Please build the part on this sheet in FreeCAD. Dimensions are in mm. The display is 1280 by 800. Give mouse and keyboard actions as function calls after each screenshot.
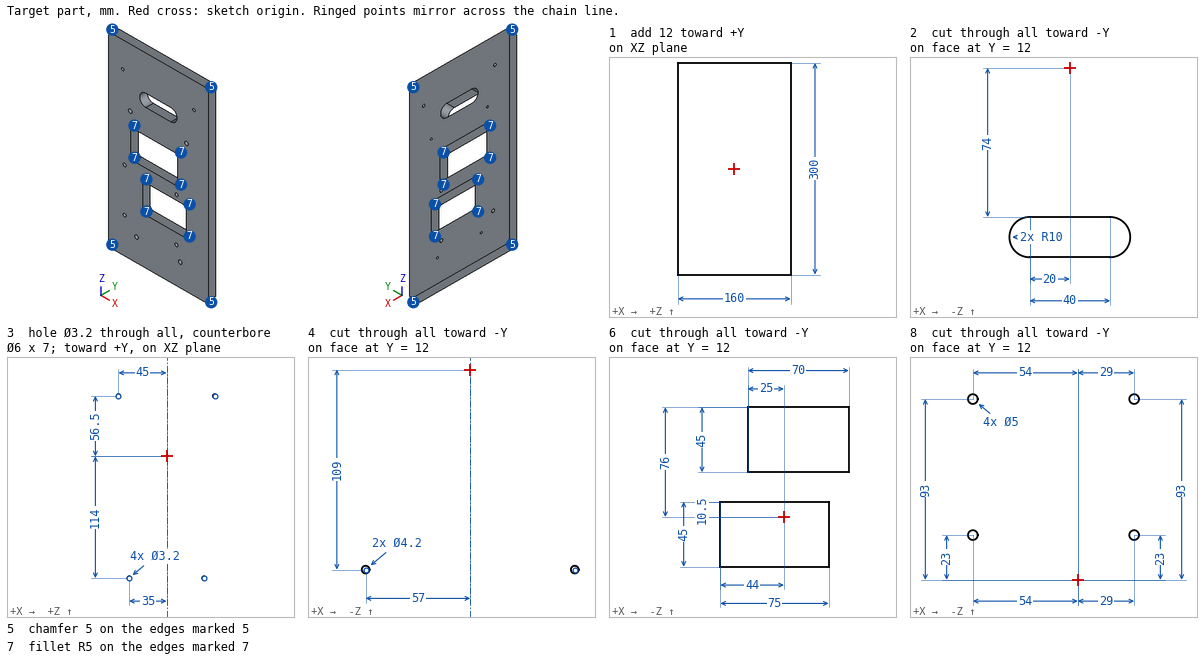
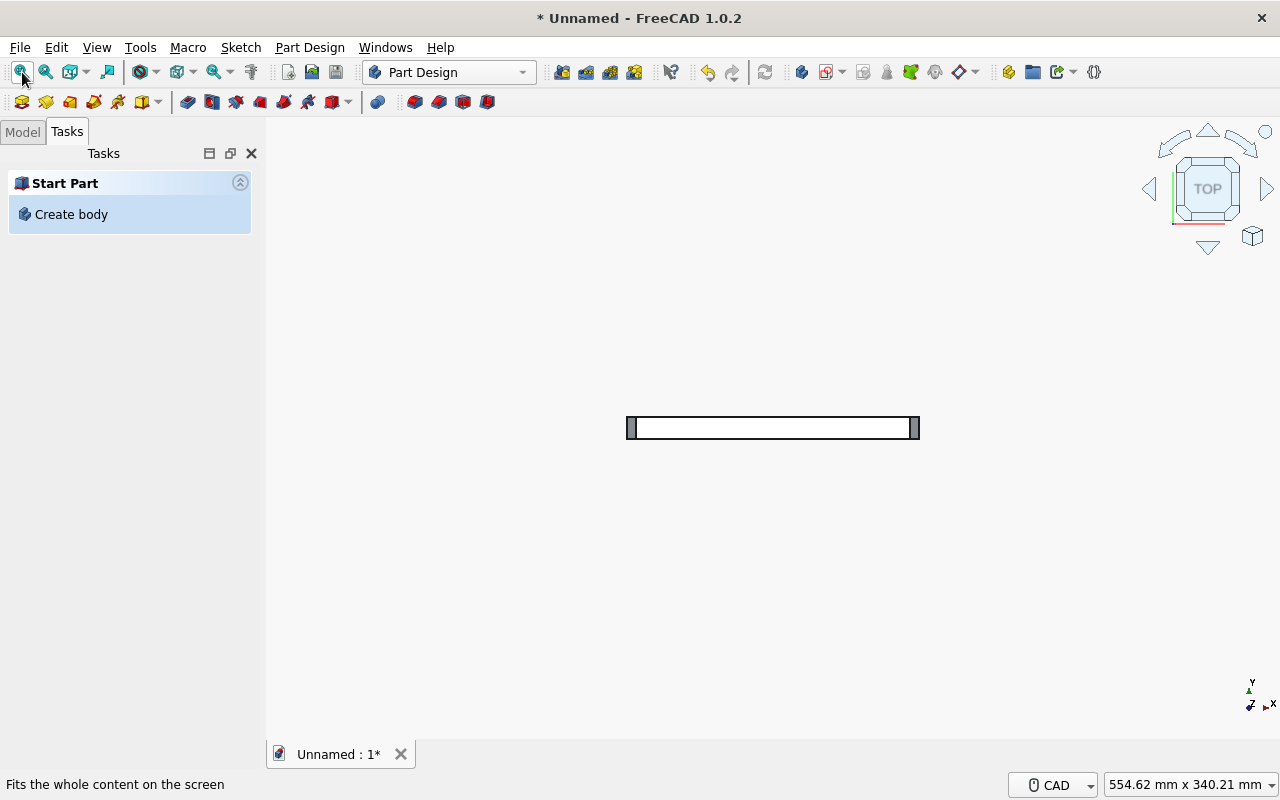
click(22, 72)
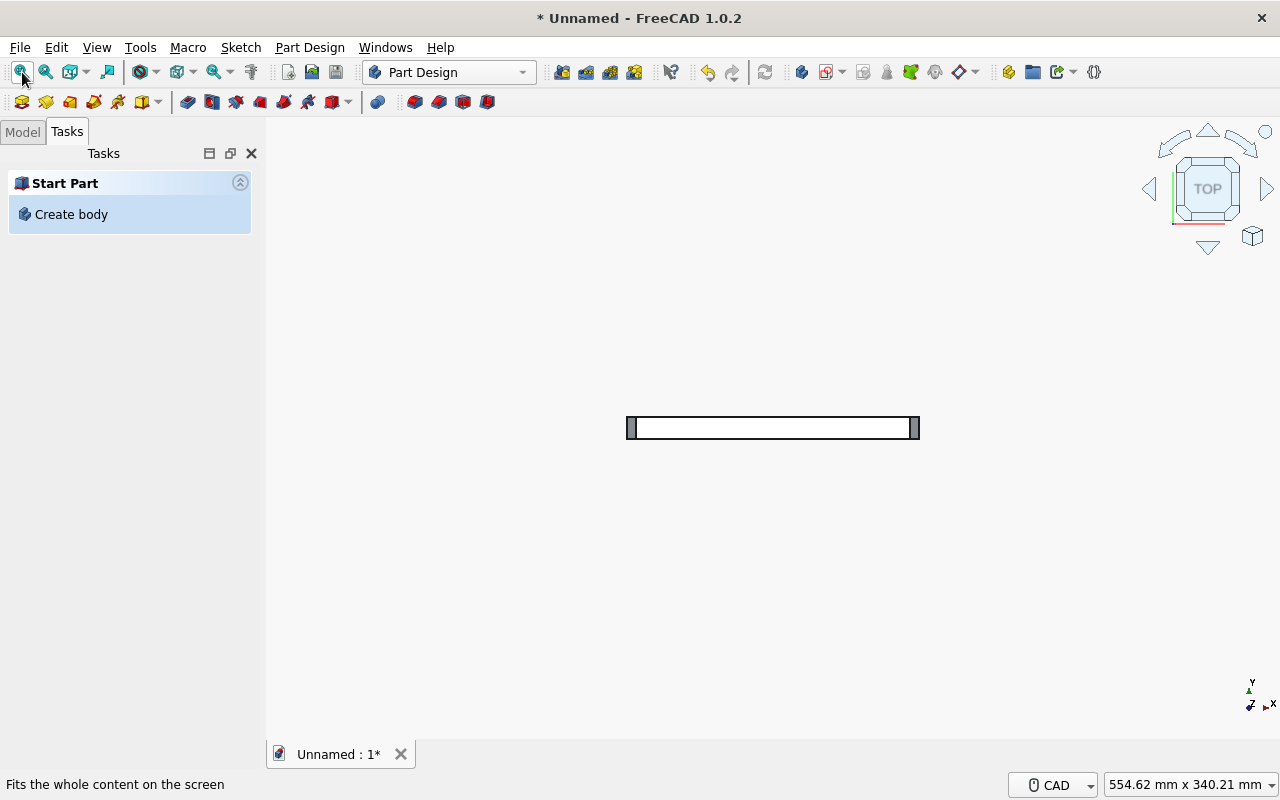
scroll(830, 427, up, 4)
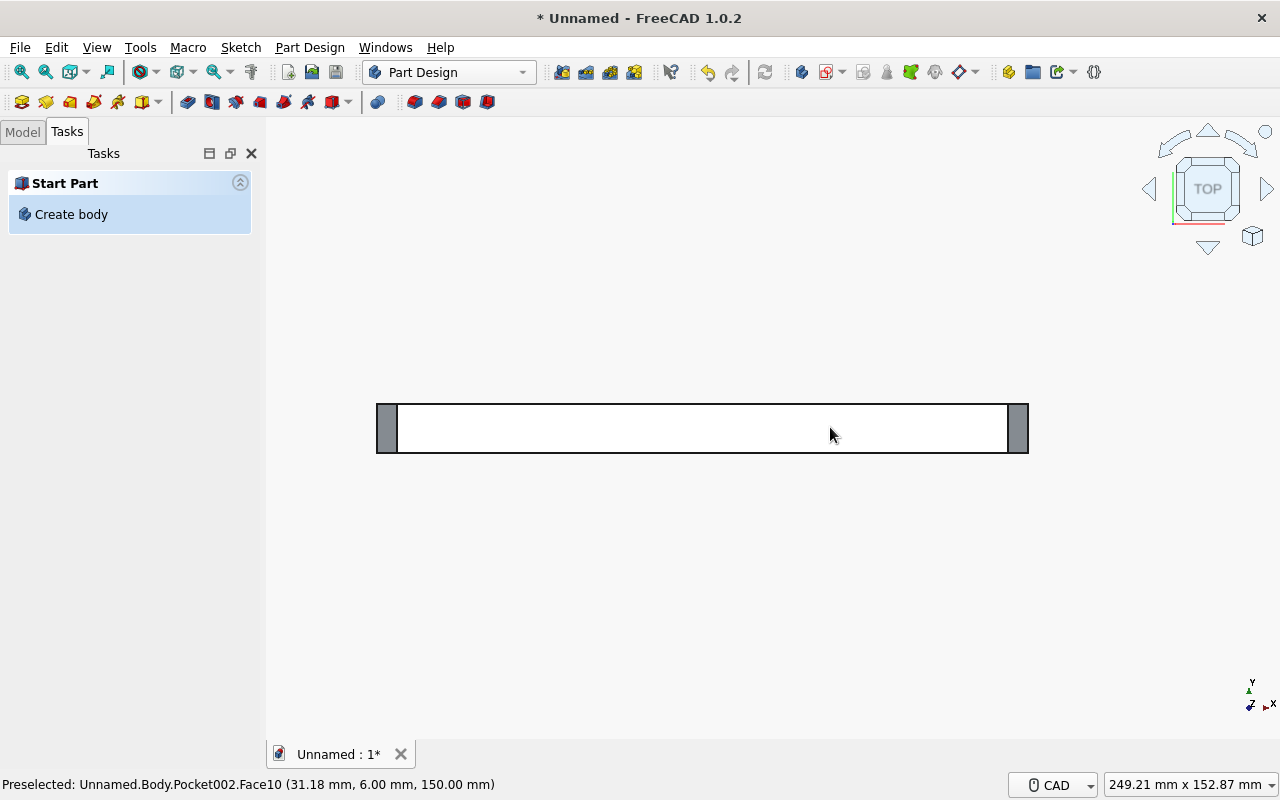
click(22, 72)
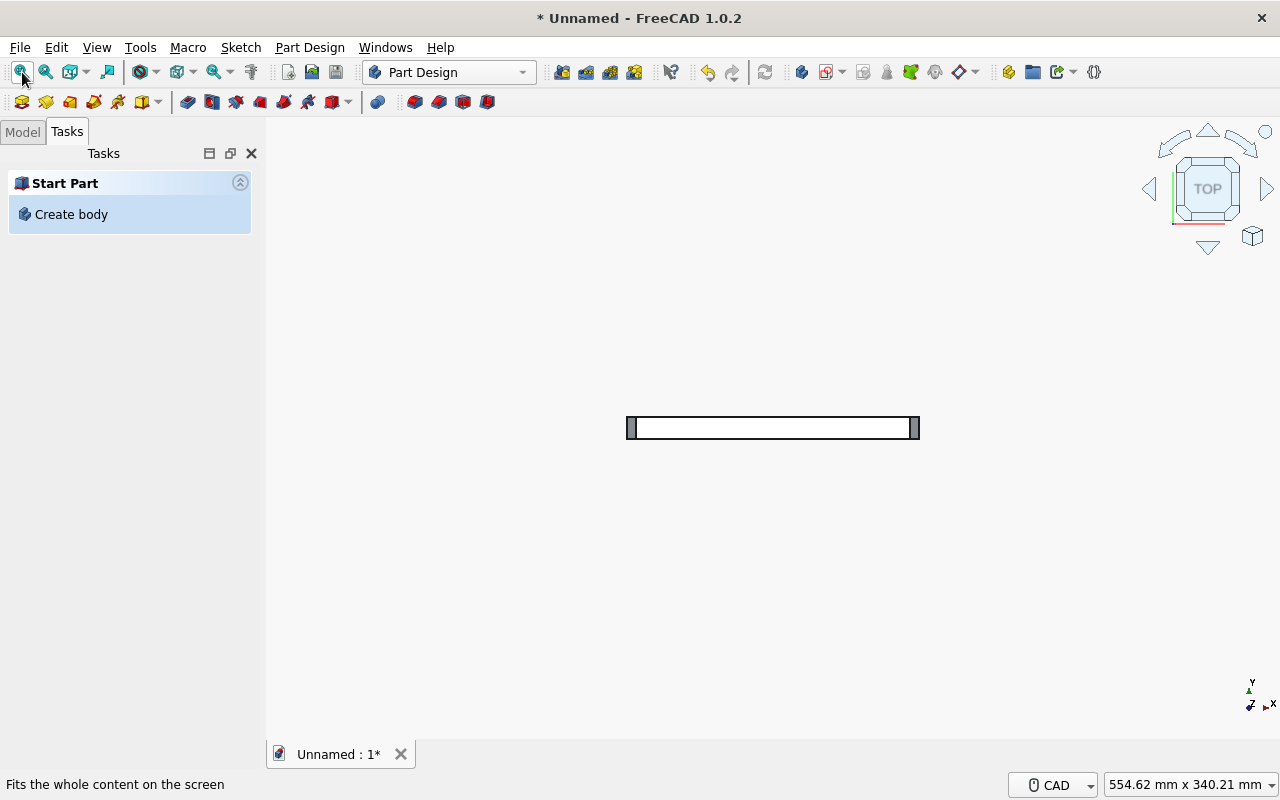
key(1)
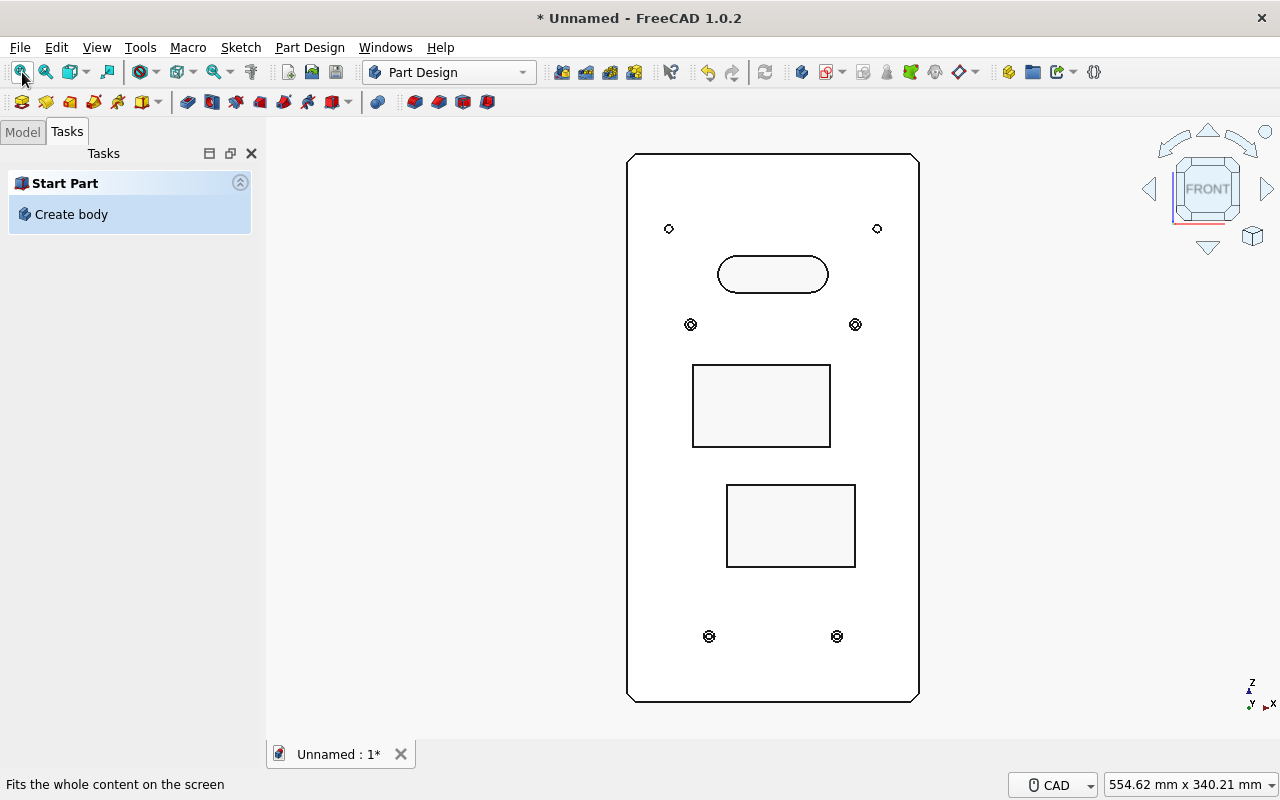
scroll(830, 446, up, 4)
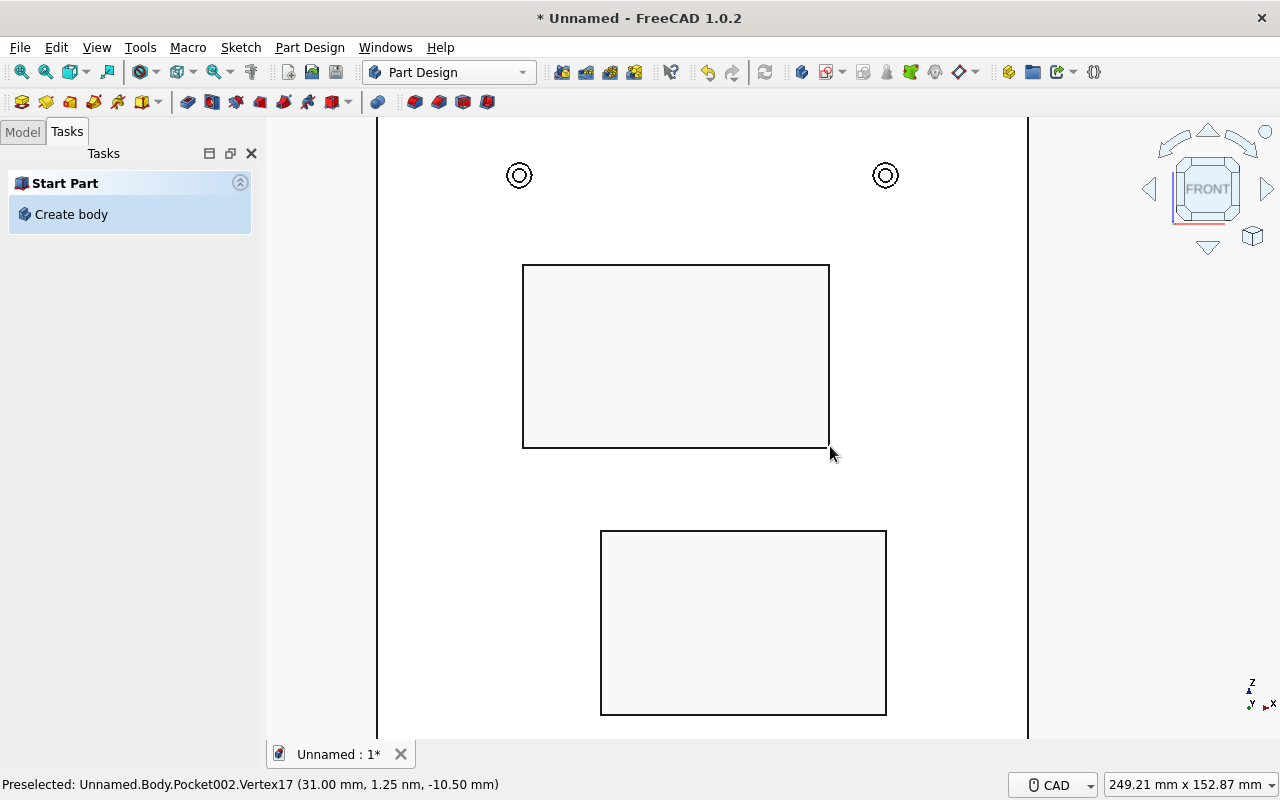
click(22, 72)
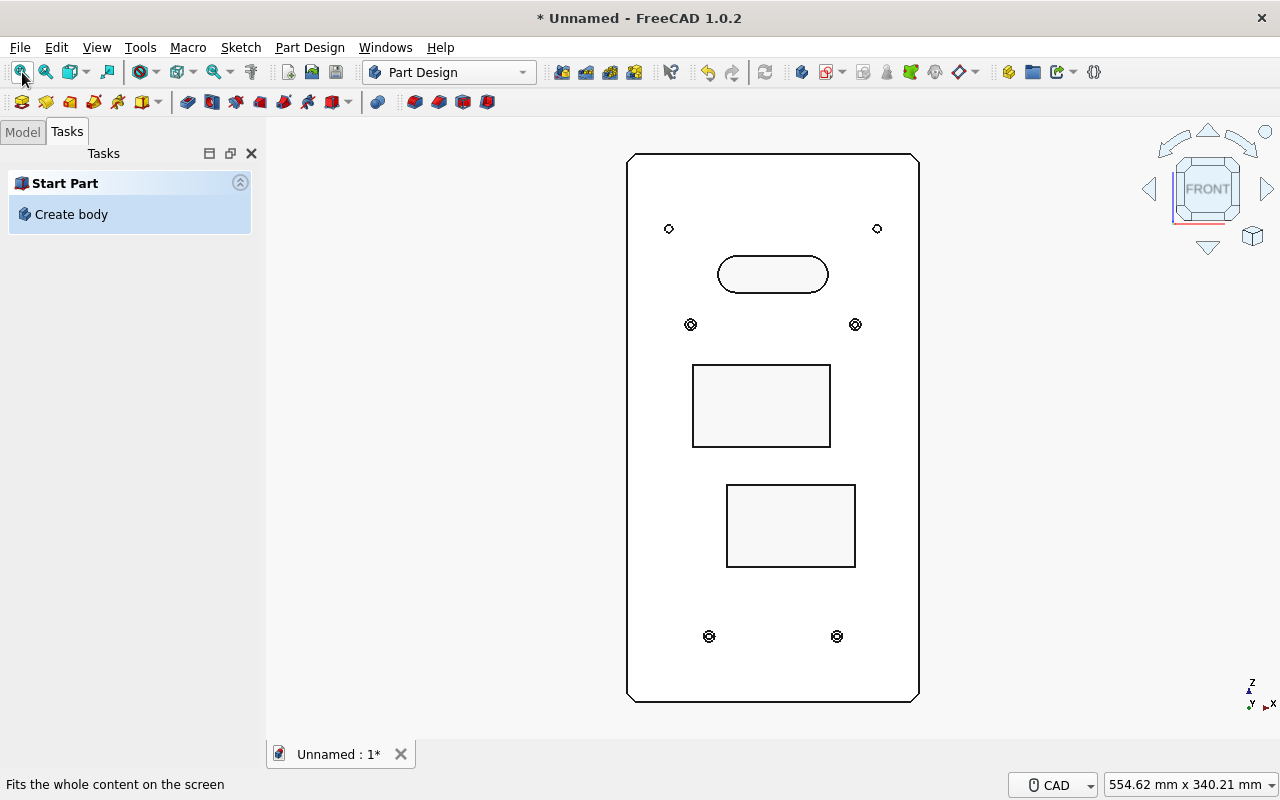
key(3)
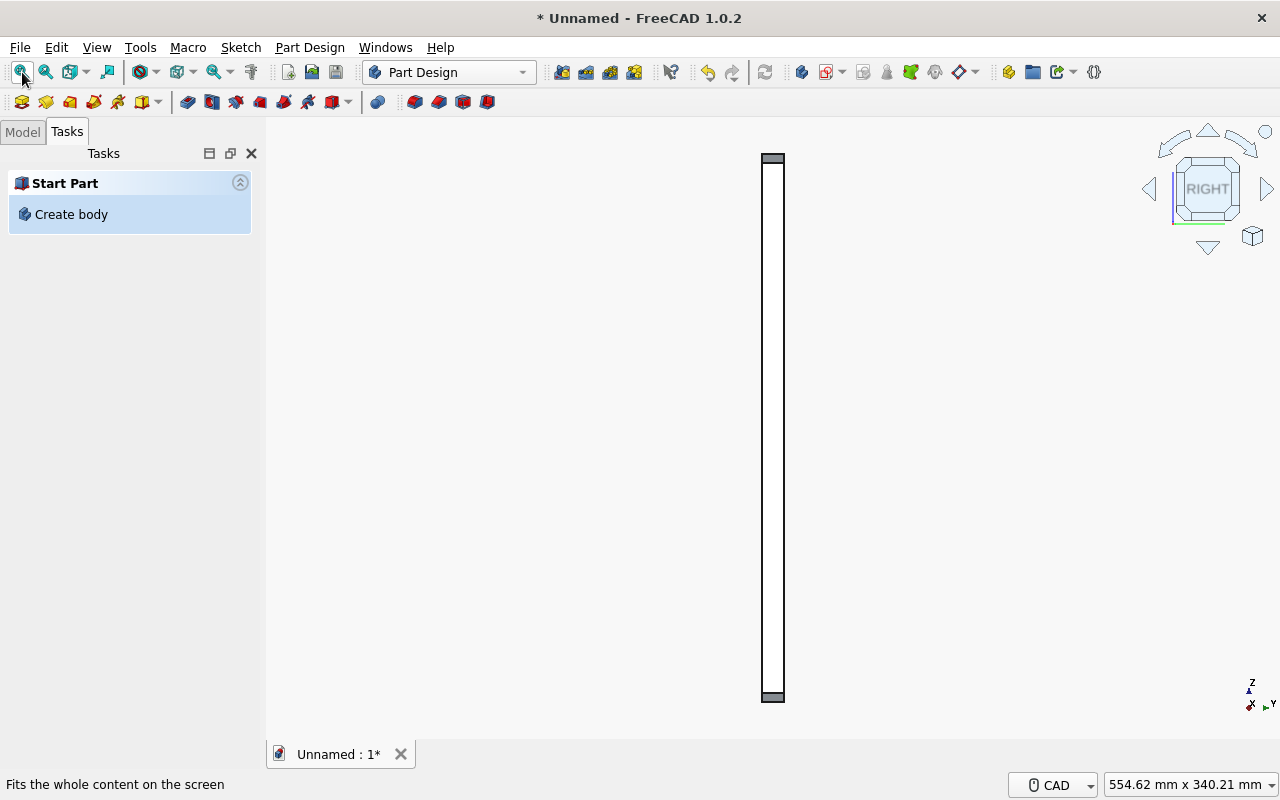
scroll(773, 446, up, 4)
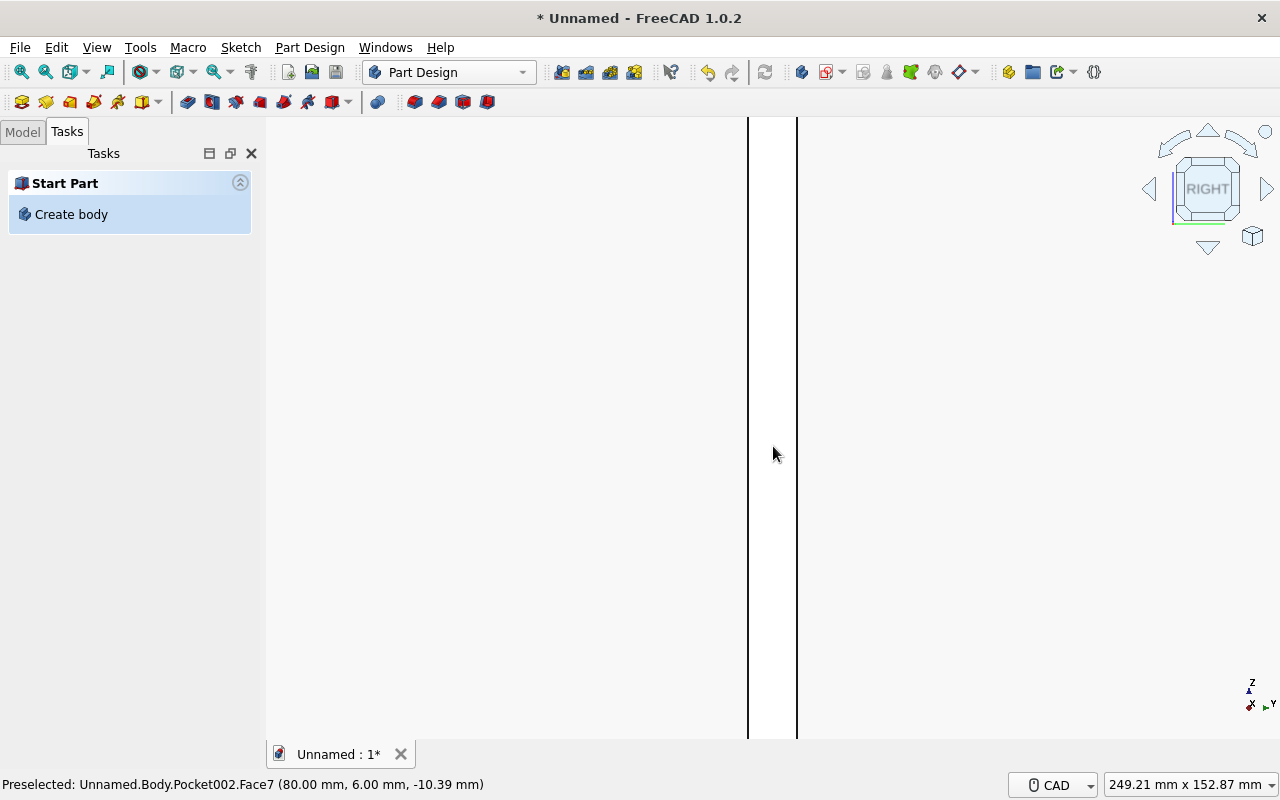
click(22, 72)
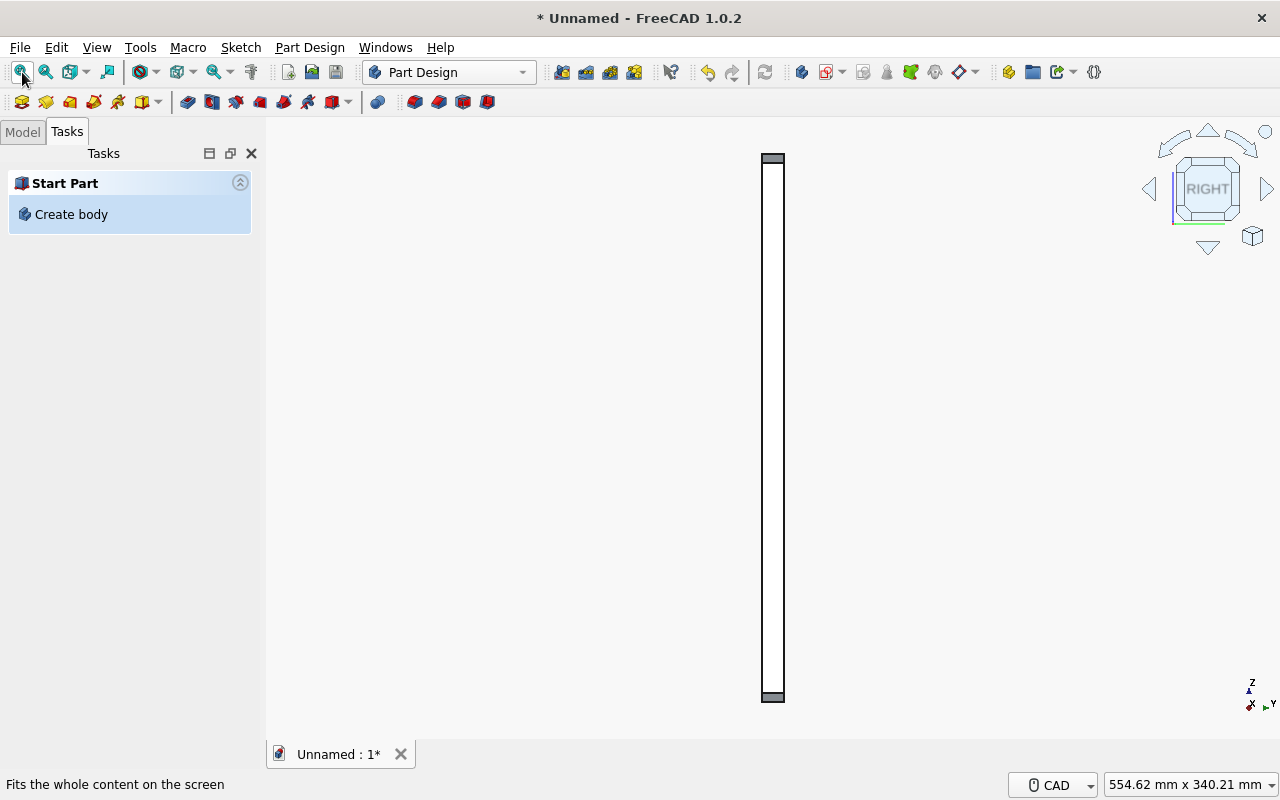
key(5)